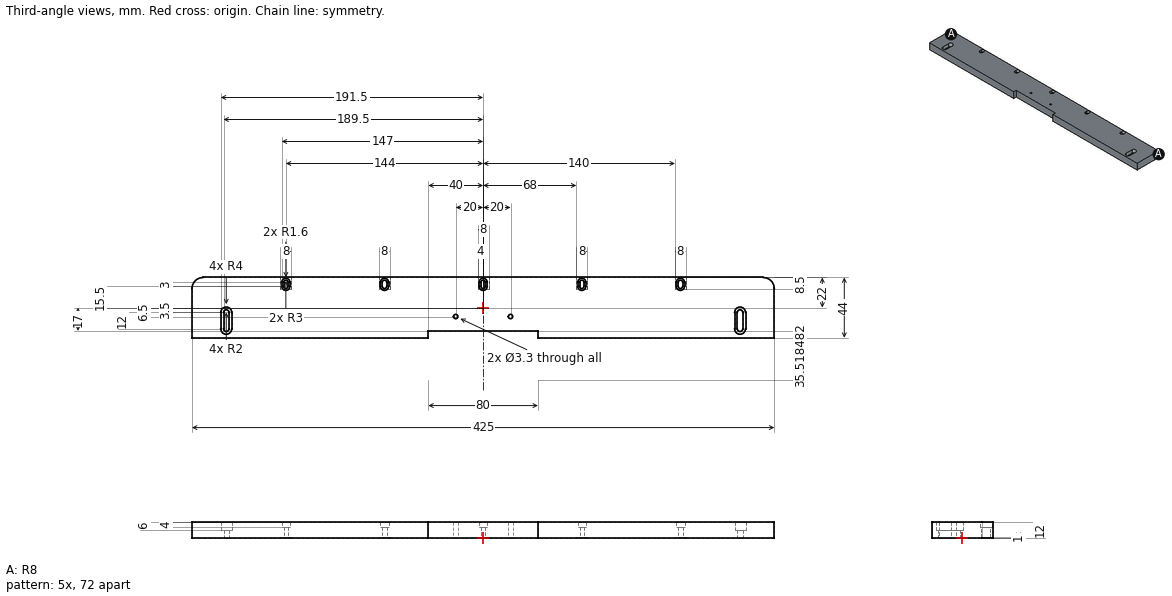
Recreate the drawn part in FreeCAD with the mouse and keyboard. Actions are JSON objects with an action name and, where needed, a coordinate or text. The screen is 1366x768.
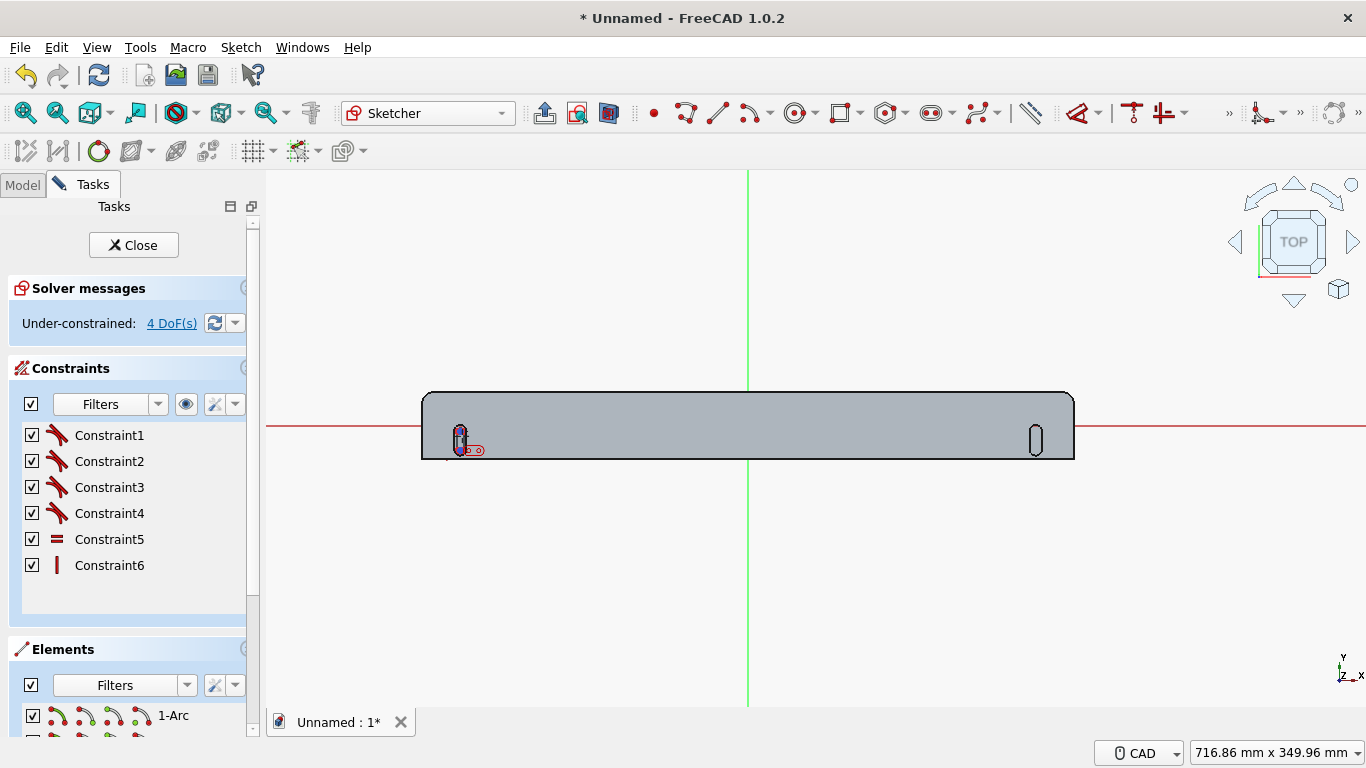
{"action": "scroll", "coordinate": [1036, 449], "scroll_direction": "up", "scroll_amount": 11}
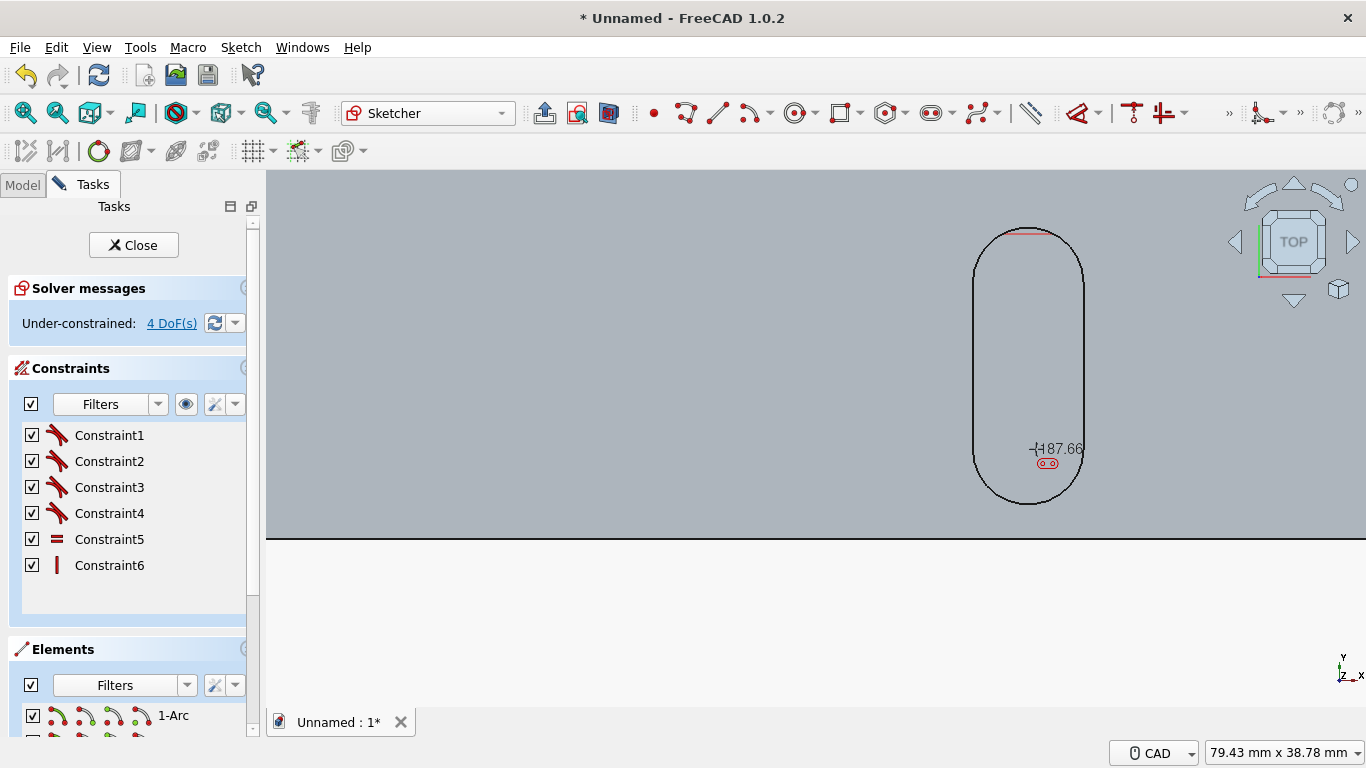
{"action": "scroll", "coordinate": [1036, 449], "scroll_direction": "down", "scroll_amount": 11}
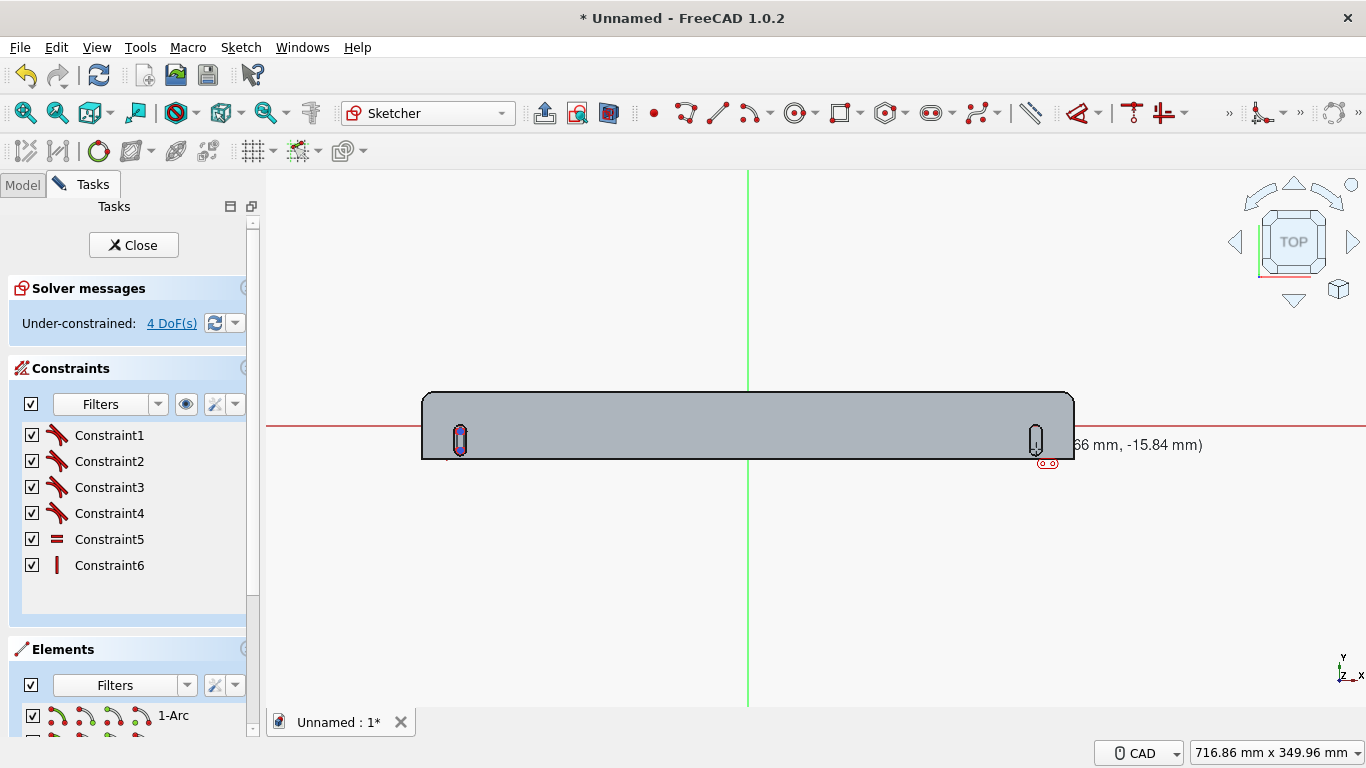
{"action": "left_click", "coordinate": [1036, 449]}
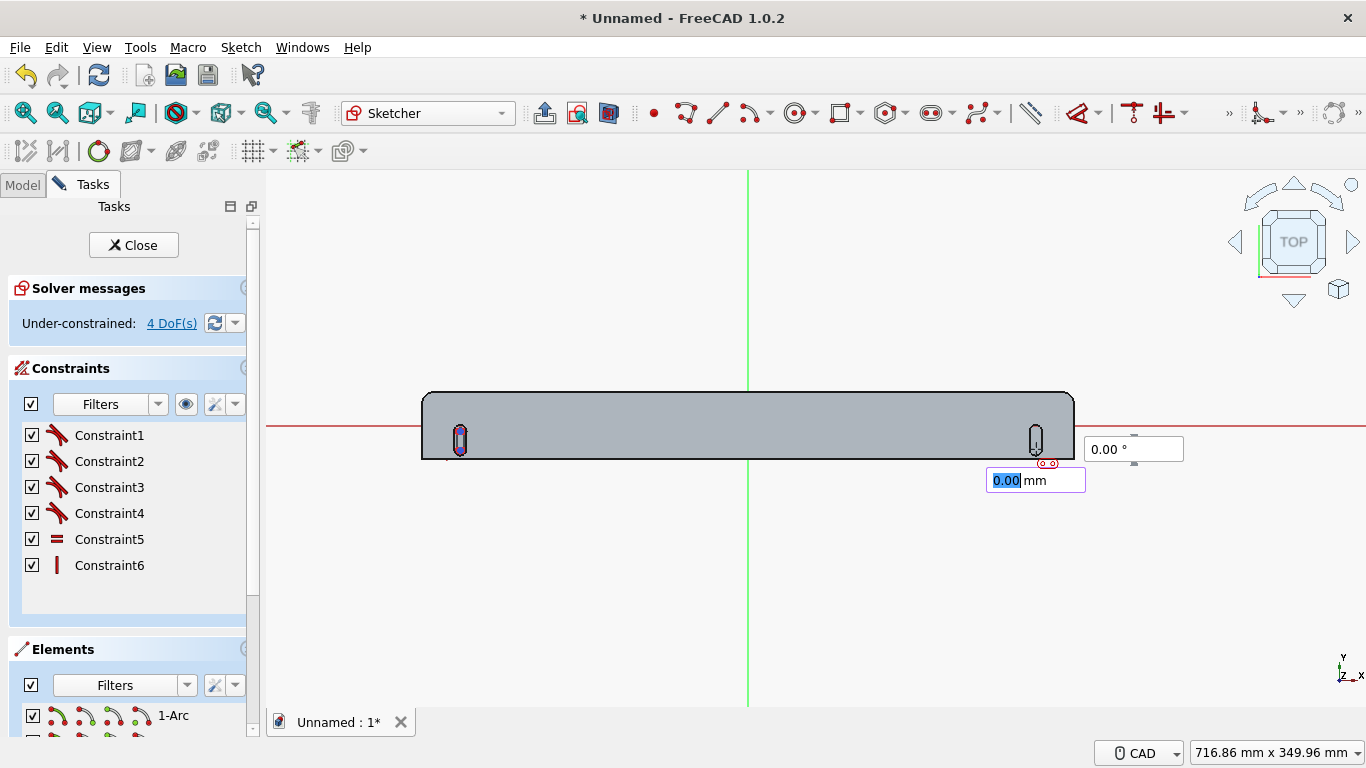
{"action": "scroll", "coordinate": [1036, 431], "scroll_direction": "up", "scroll_amount": 6}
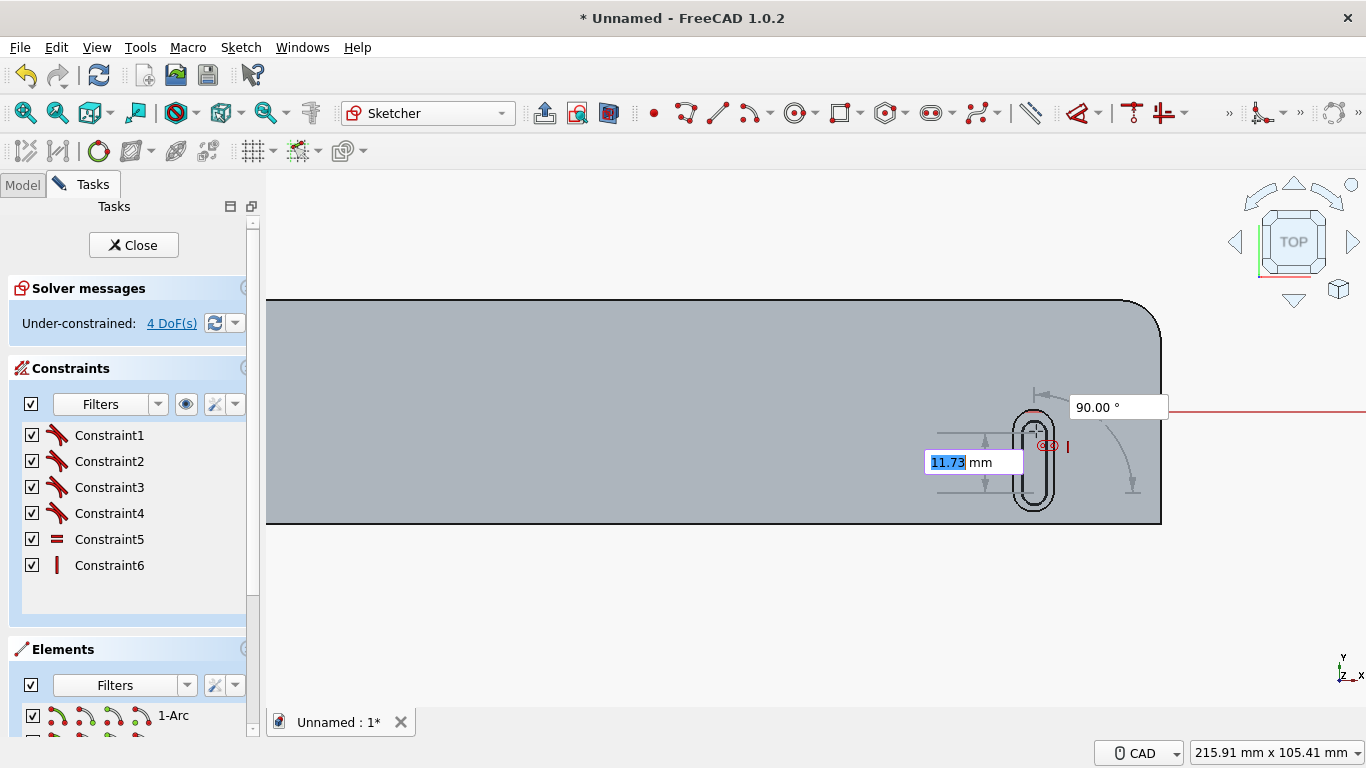
{"action": "left_click", "coordinate": [1034, 430]}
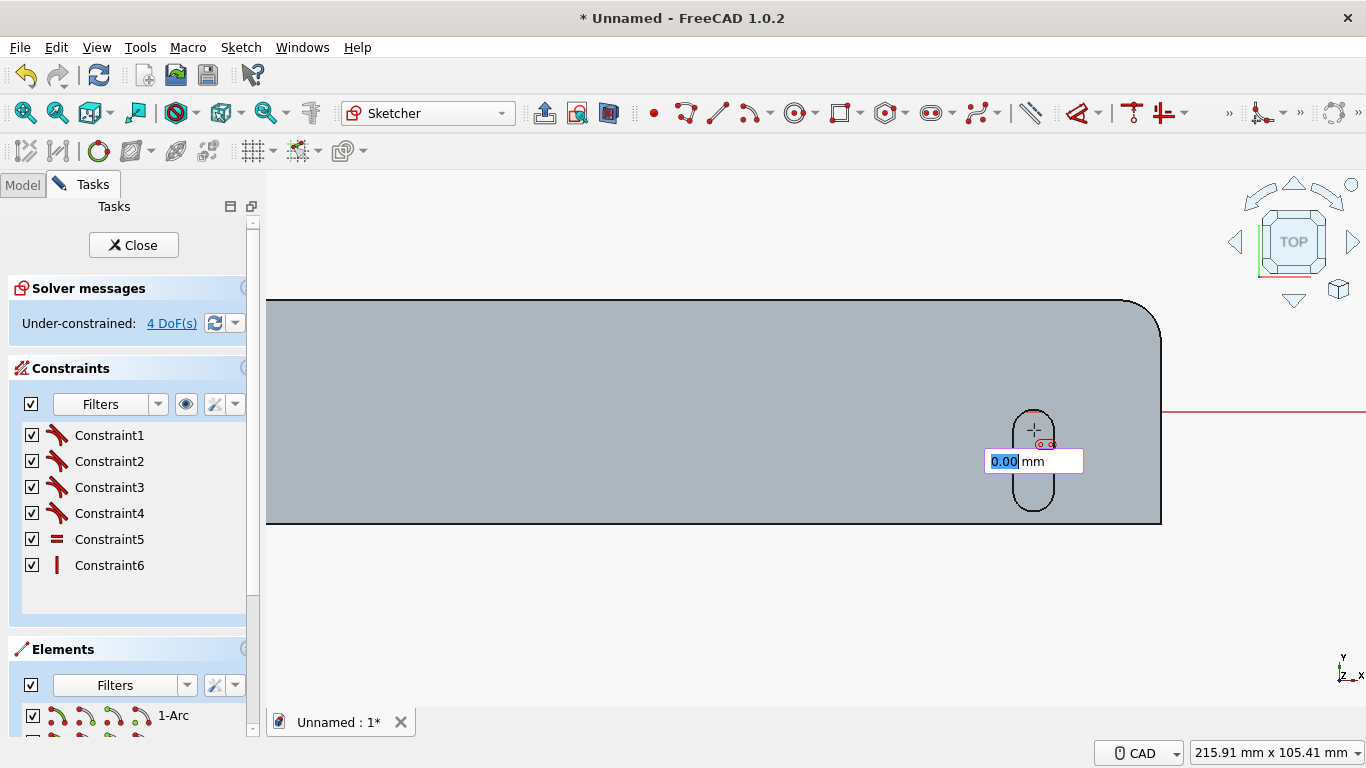
{"action": "scroll", "coordinate": [1044, 461], "scroll_direction": "up", "scroll_amount": 3}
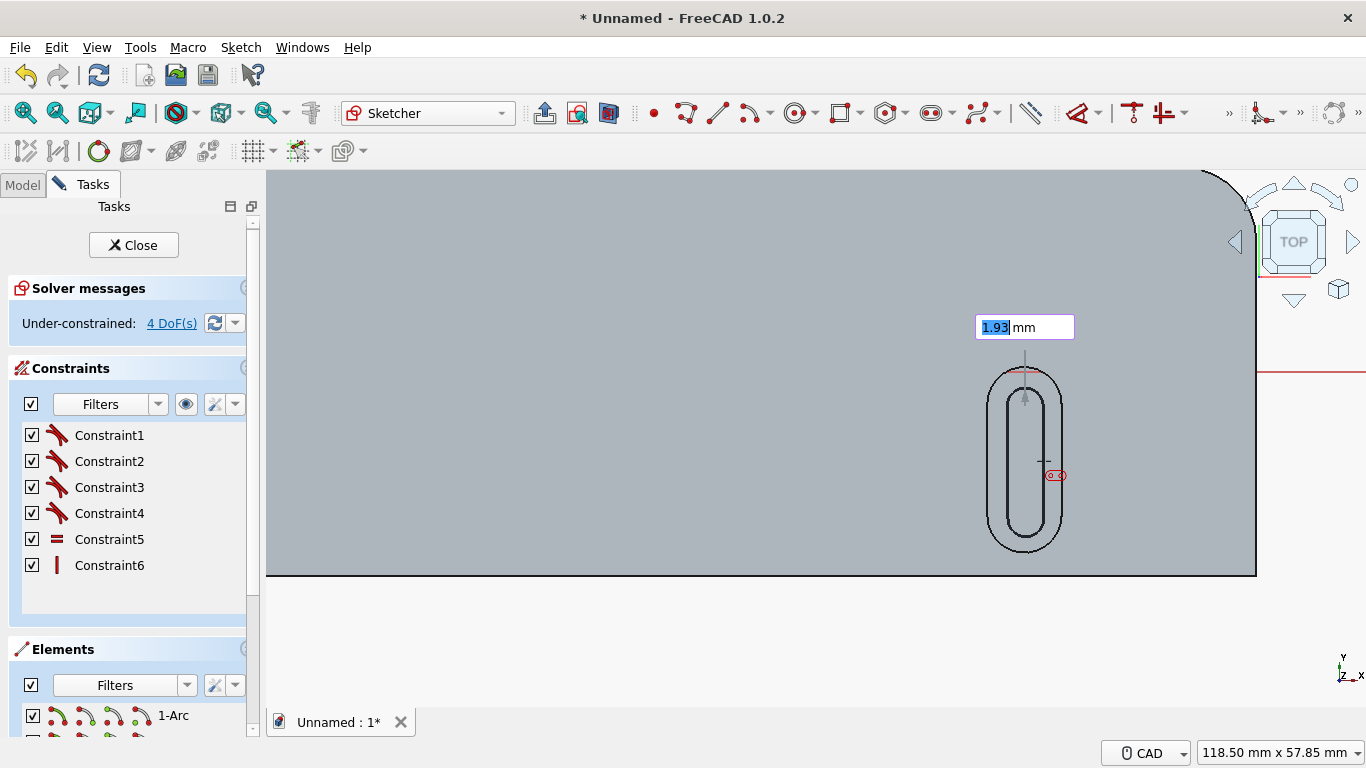
{"action": "left_click", "coordinate": [1043, 460]}
{"action": "key", "text": "Escape"}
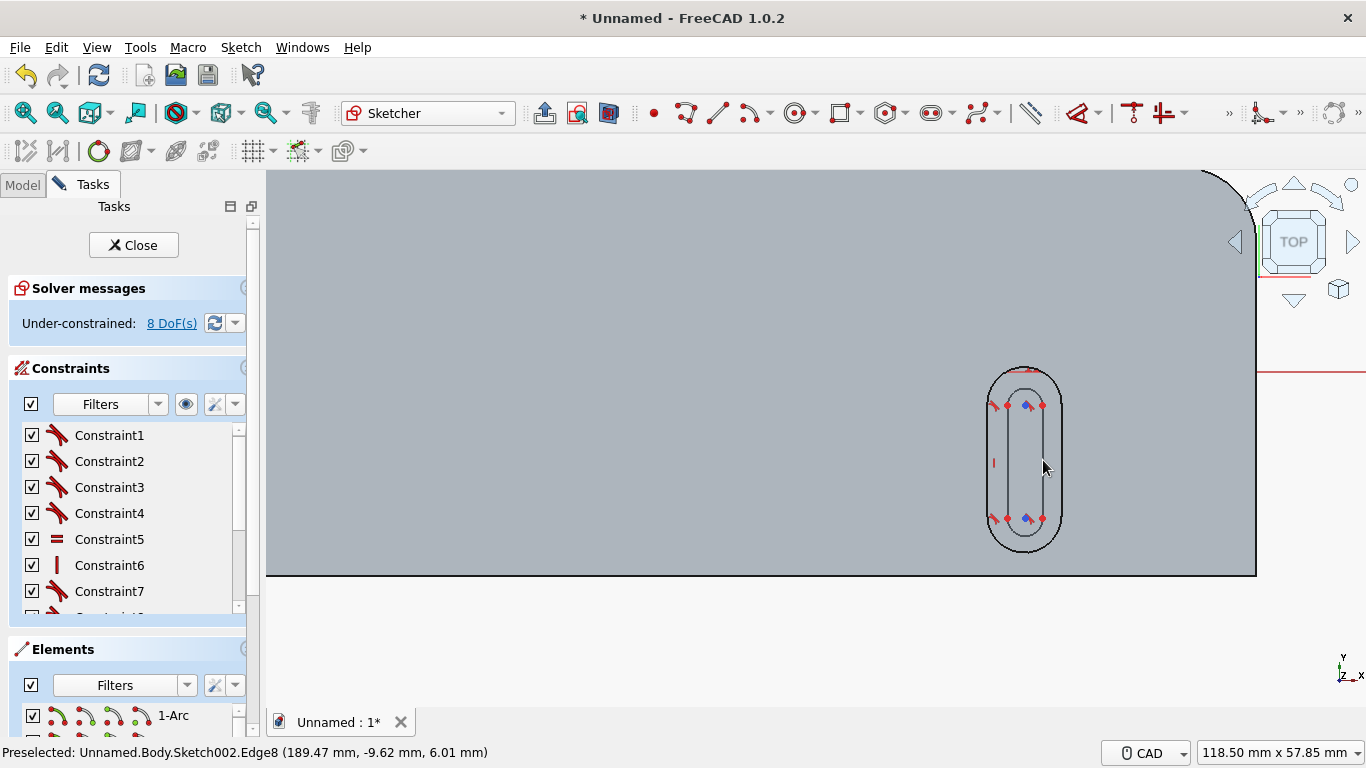
{"action": "scroll", "coordinate": [1037, 436], "scroll_direction": "down", "scroll_amount": 9}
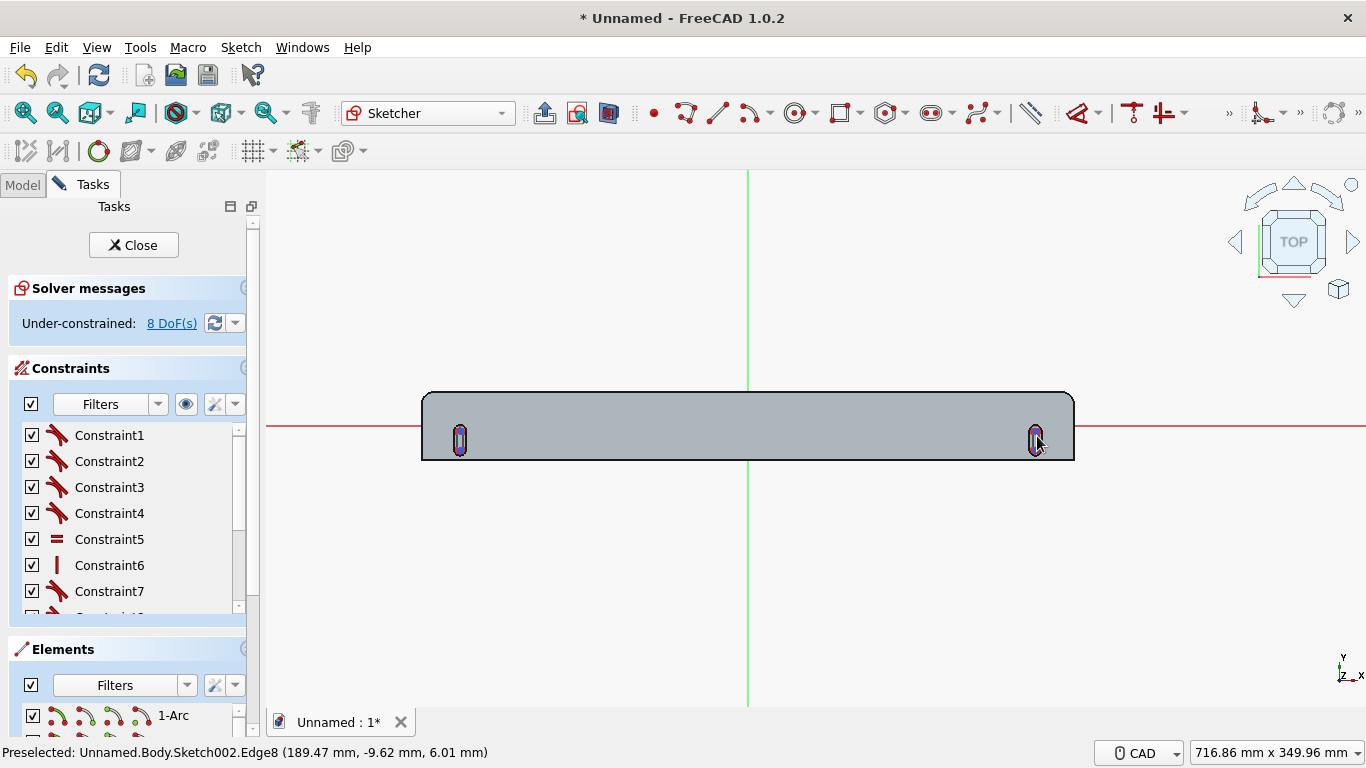
{"action": "scroll", "coordinate": [458, 453], "scroll_direction": "up", "scroll_amount": 8}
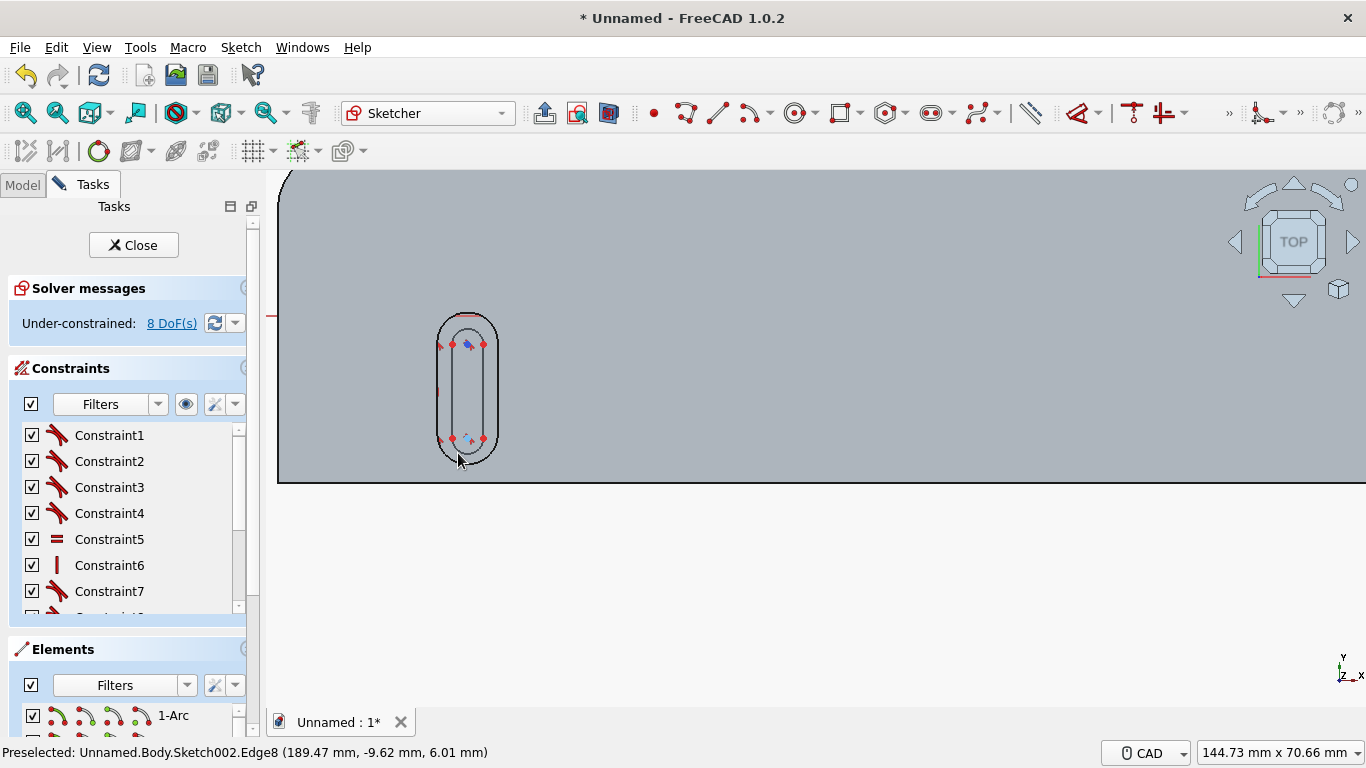
{"action": "left_click", "coordinate": [459, 451]}